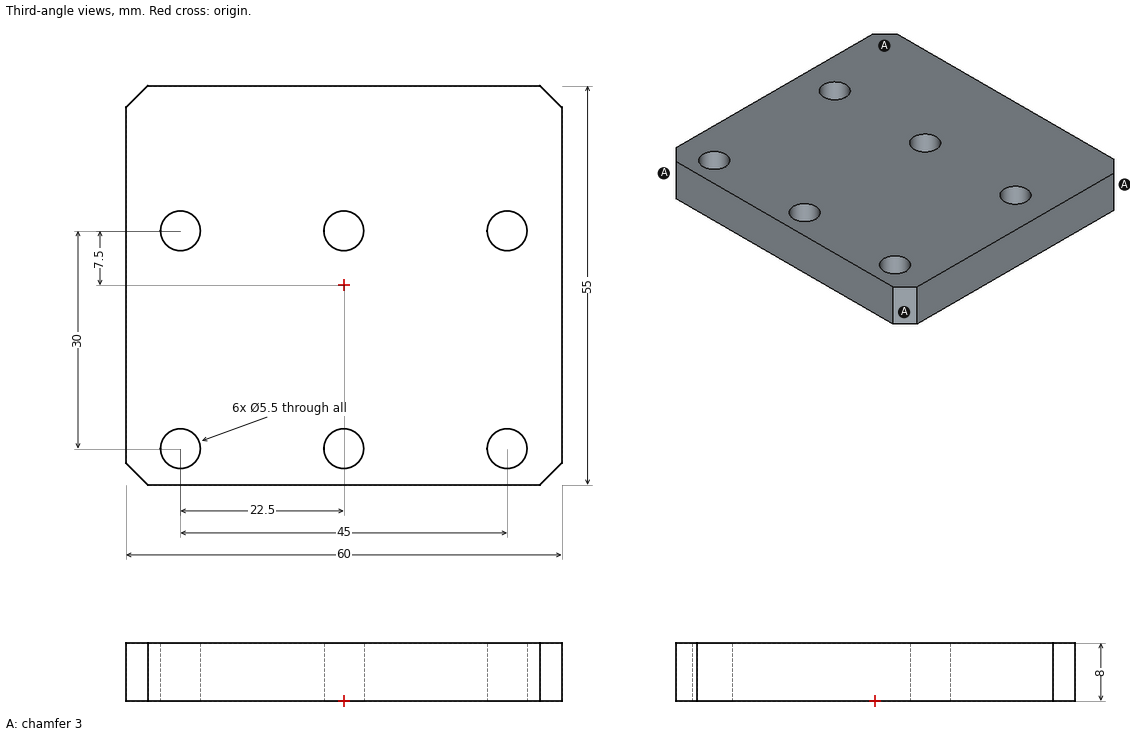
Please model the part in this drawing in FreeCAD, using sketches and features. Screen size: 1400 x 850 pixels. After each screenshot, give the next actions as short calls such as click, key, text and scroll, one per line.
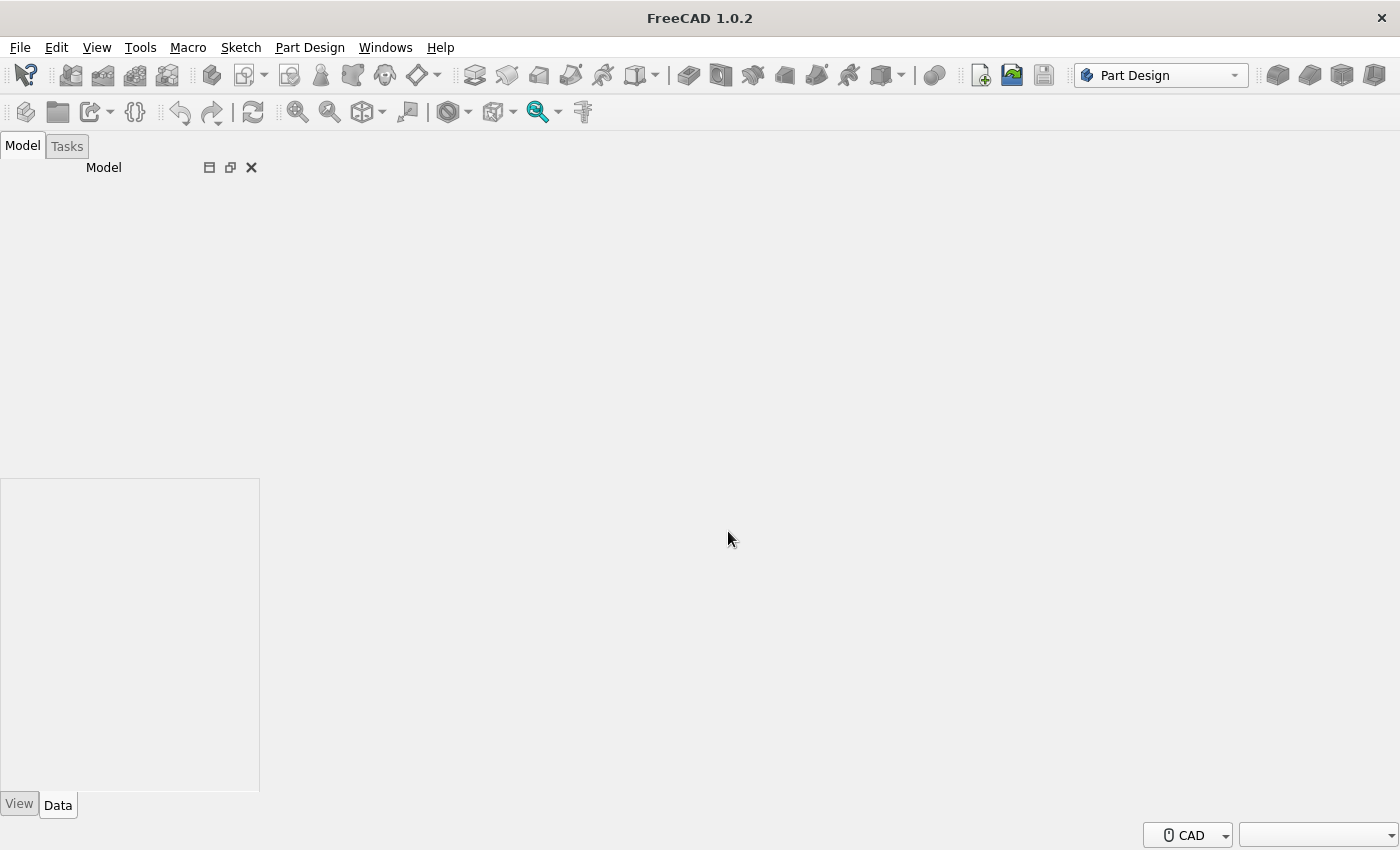
click(980, 76)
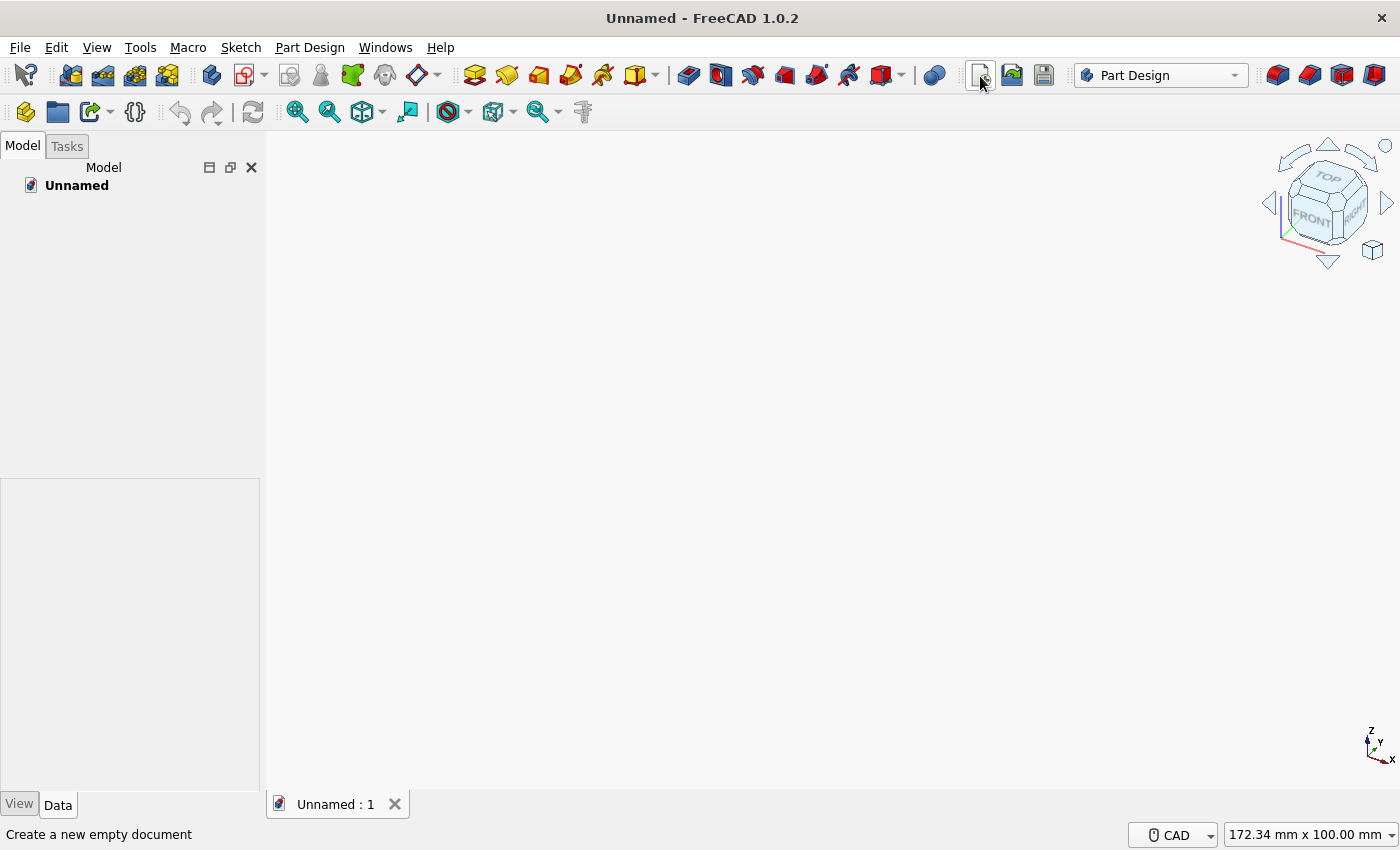
click(244, 76)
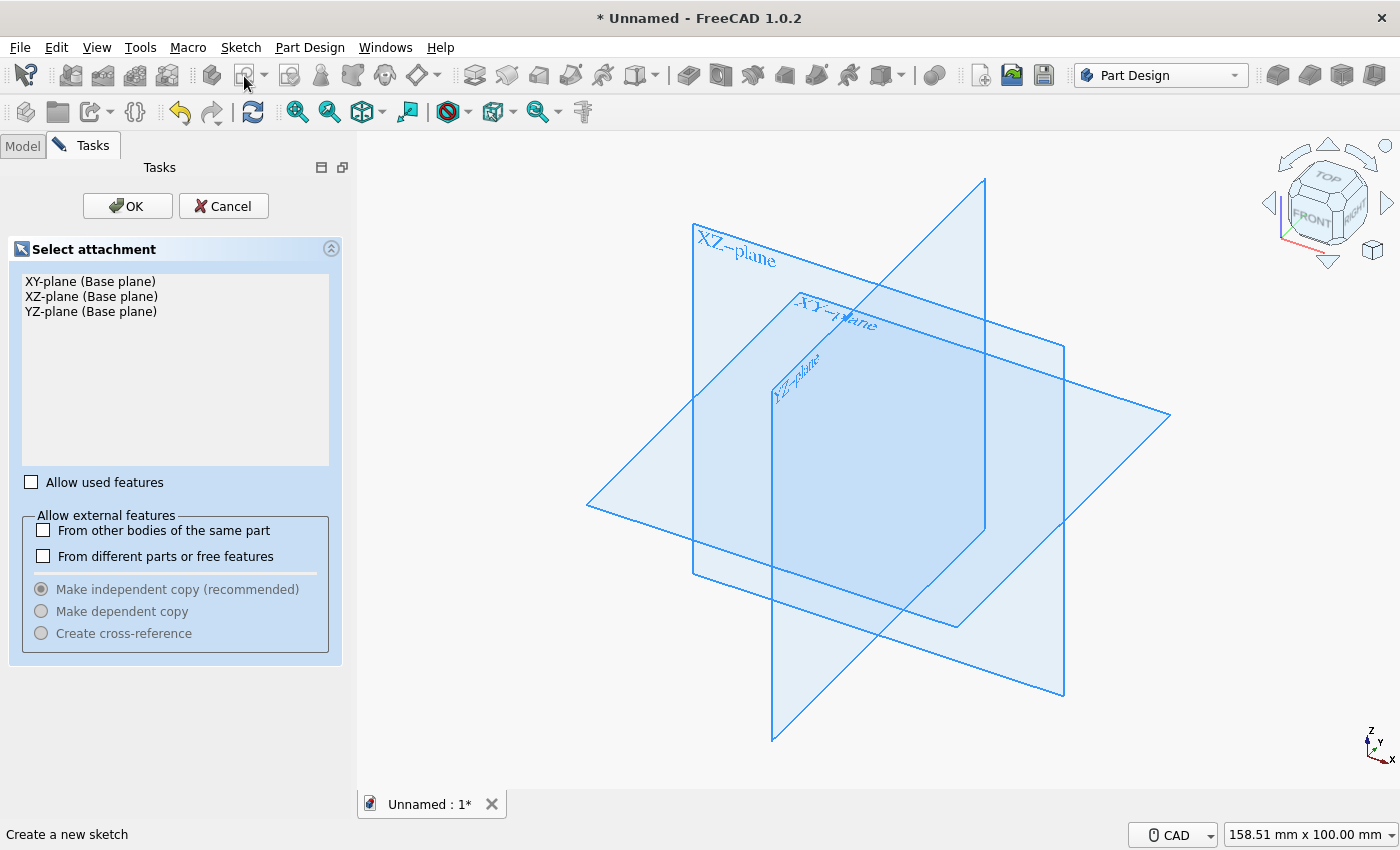
click(82, 282)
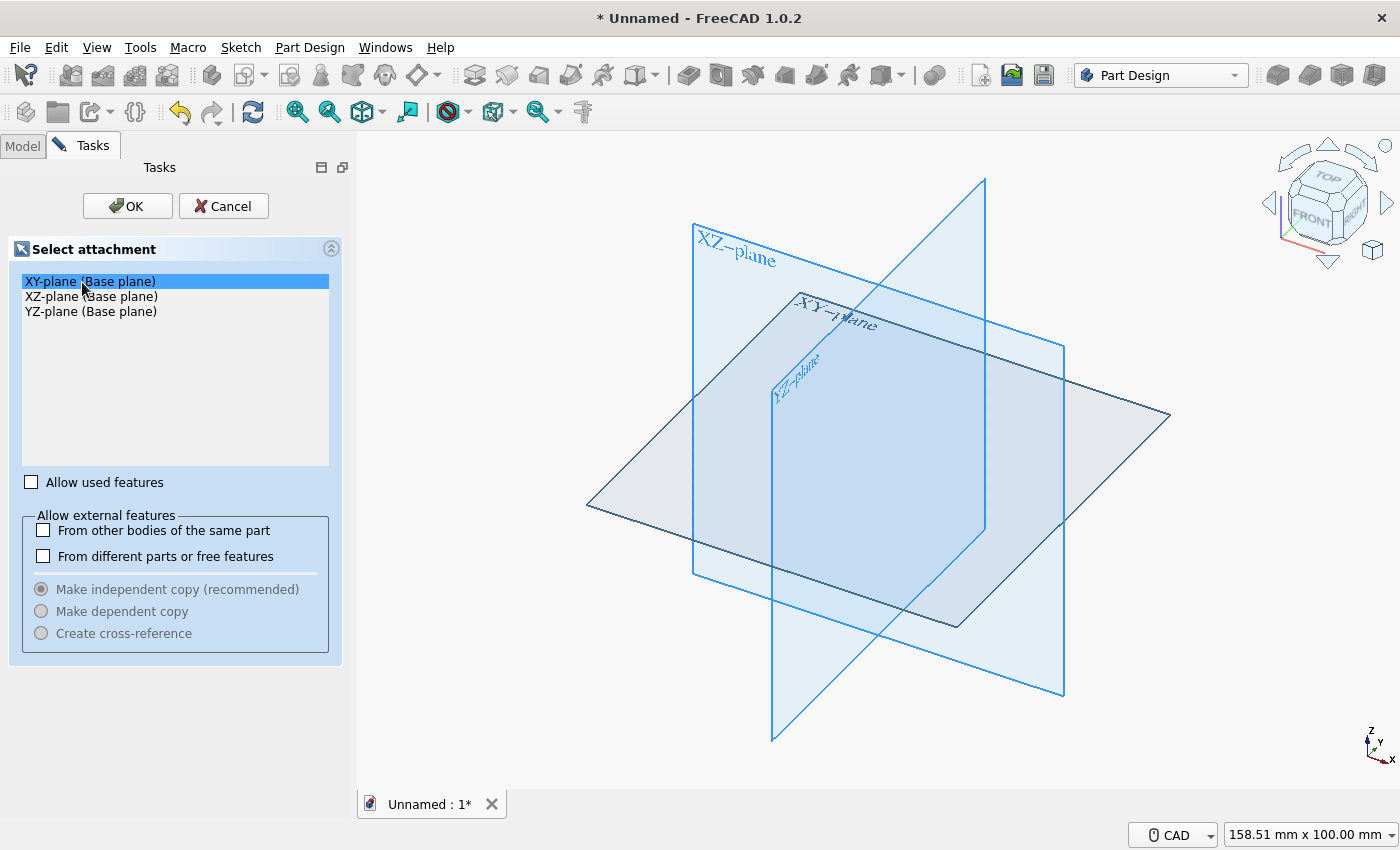
click(128, 206)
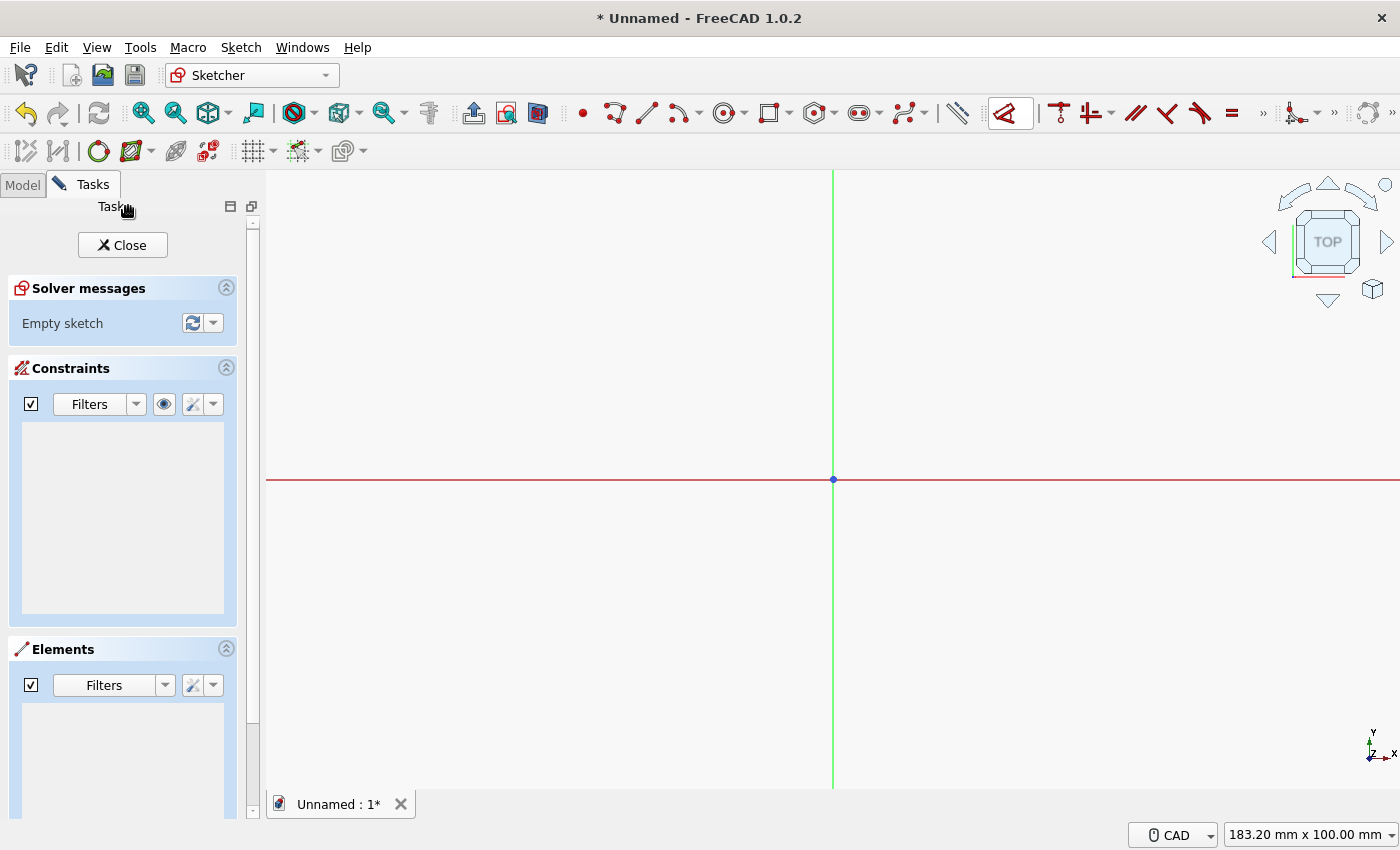
key(g)
key(v)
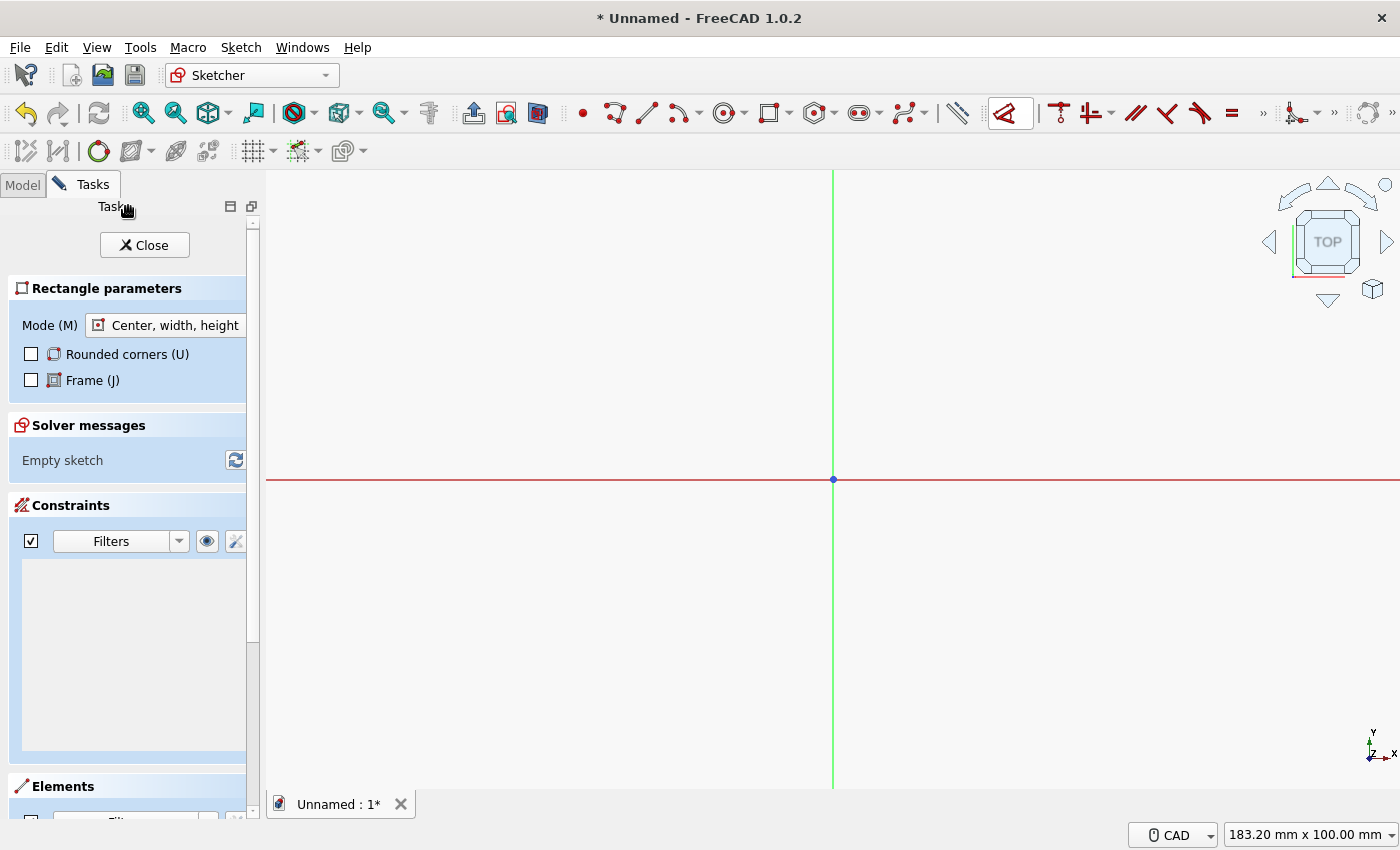
click(833, 480)
click(1019, 309)
key(Escape)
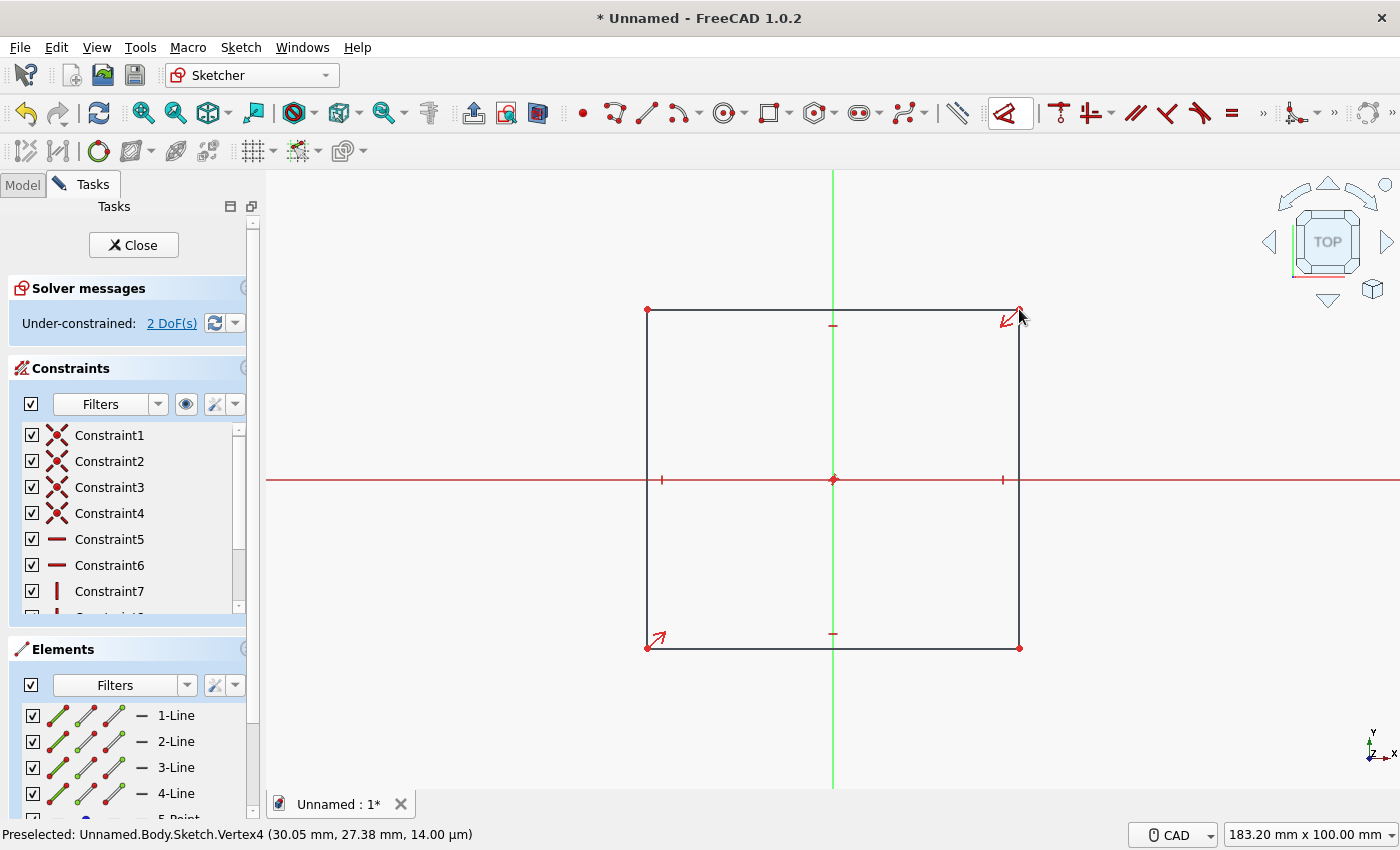
key(d)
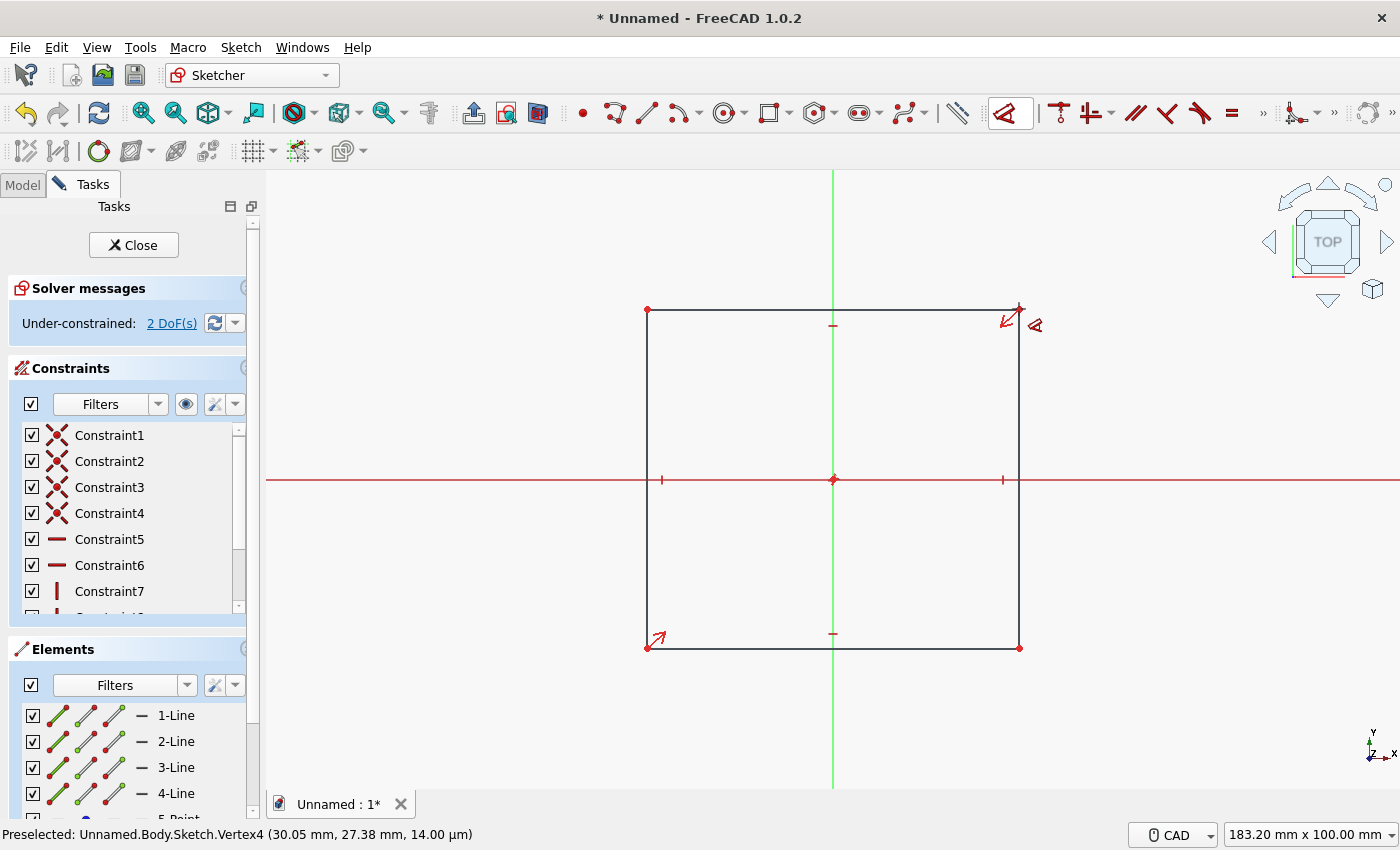
click(759, 649)
click(747, 683)